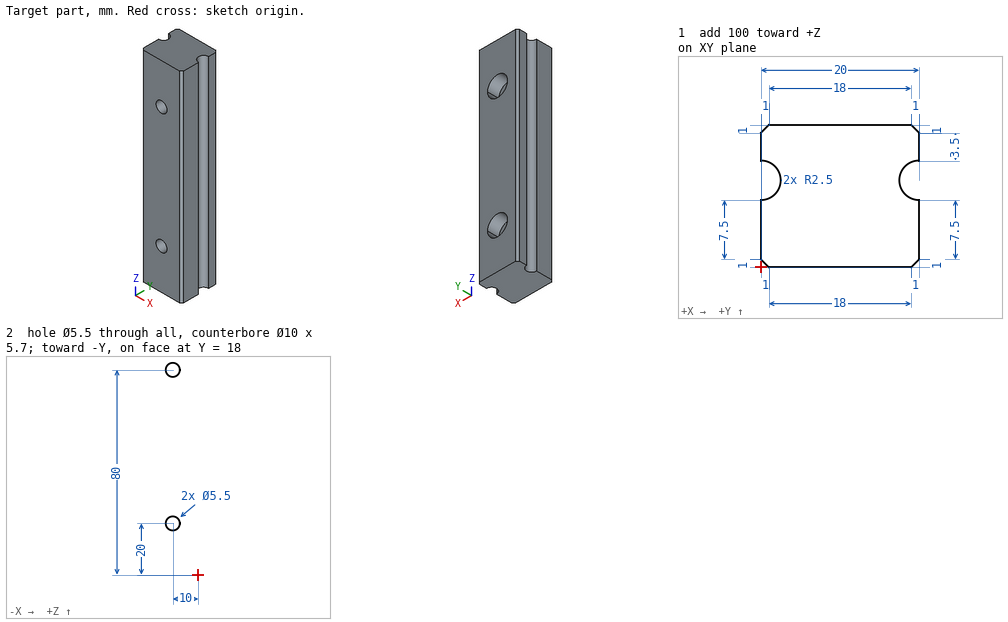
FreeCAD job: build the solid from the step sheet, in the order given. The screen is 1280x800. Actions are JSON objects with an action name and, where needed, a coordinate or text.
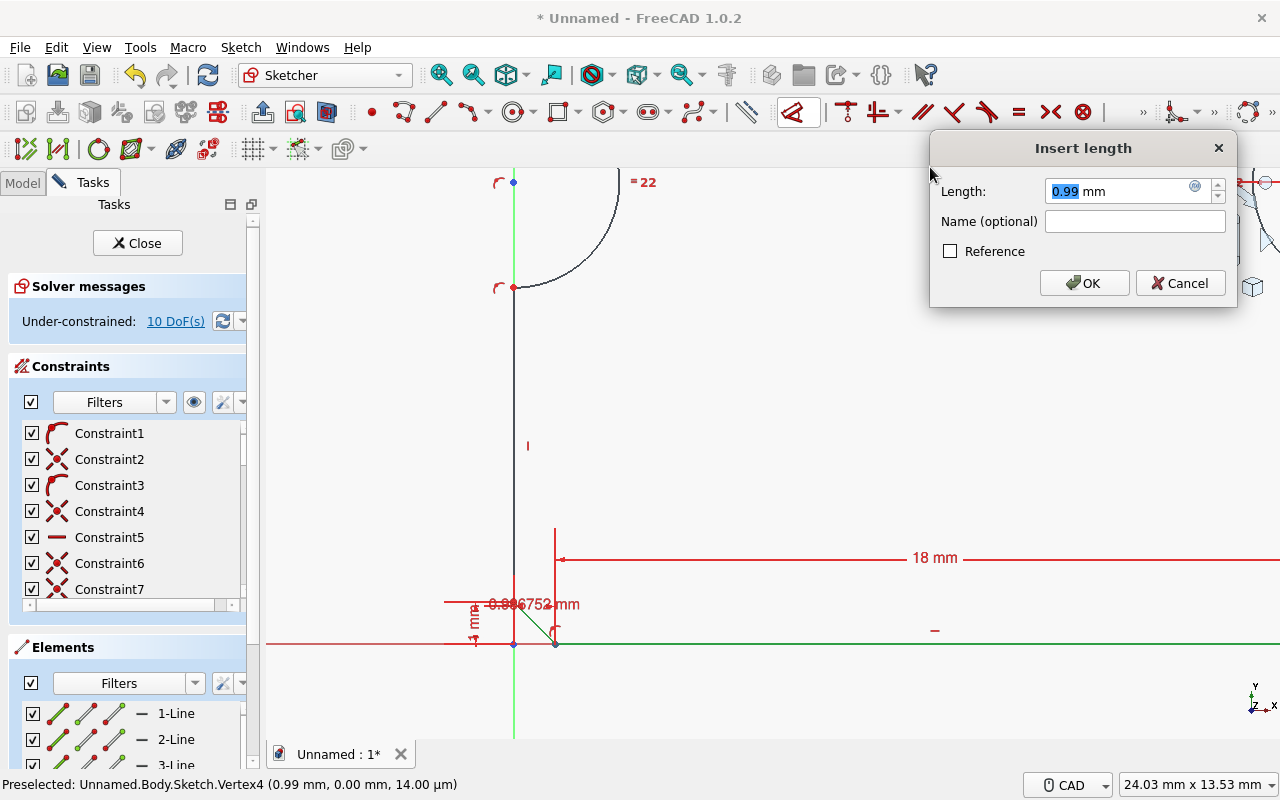
{"action": "type", "text": "1"}
{"action": "key", "text": "Return"}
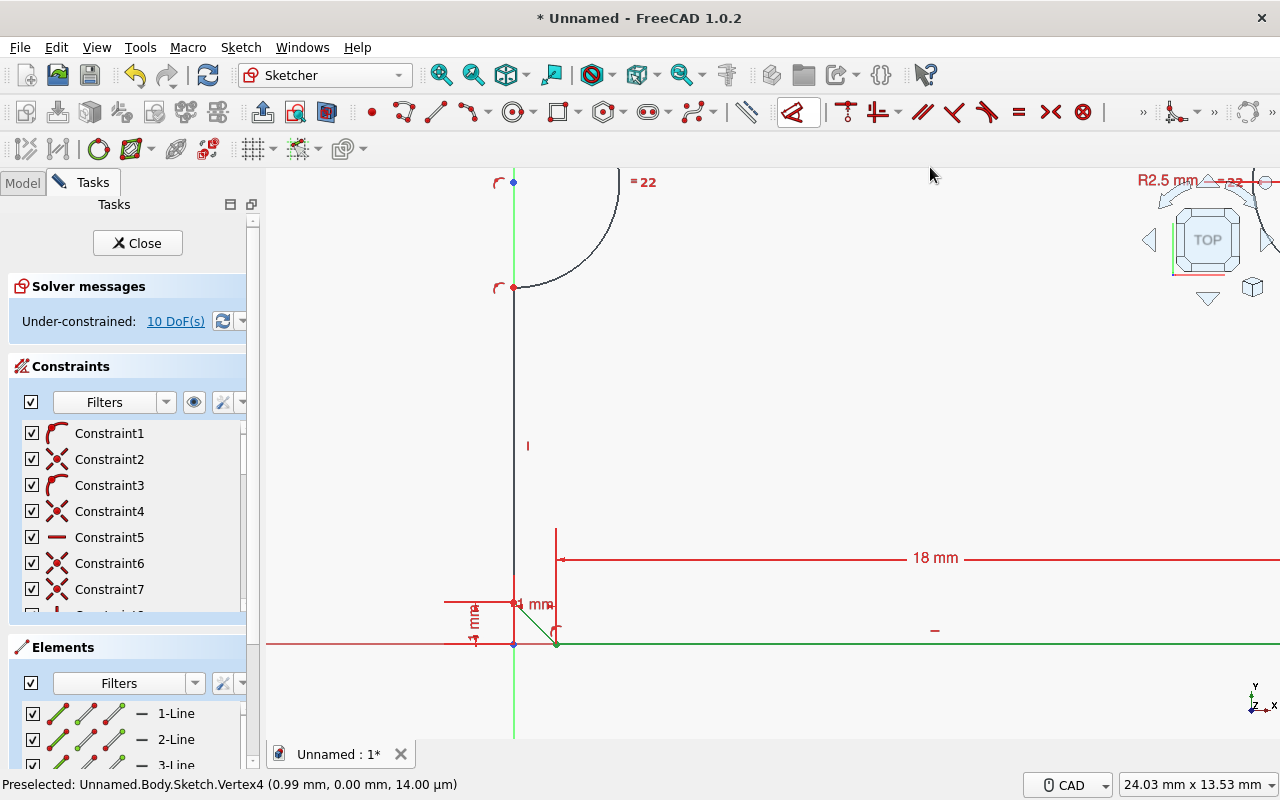
{"action": "scroll", "coordinate": [516, 608], "scroll_direction": "down", "scroll_amount": 4}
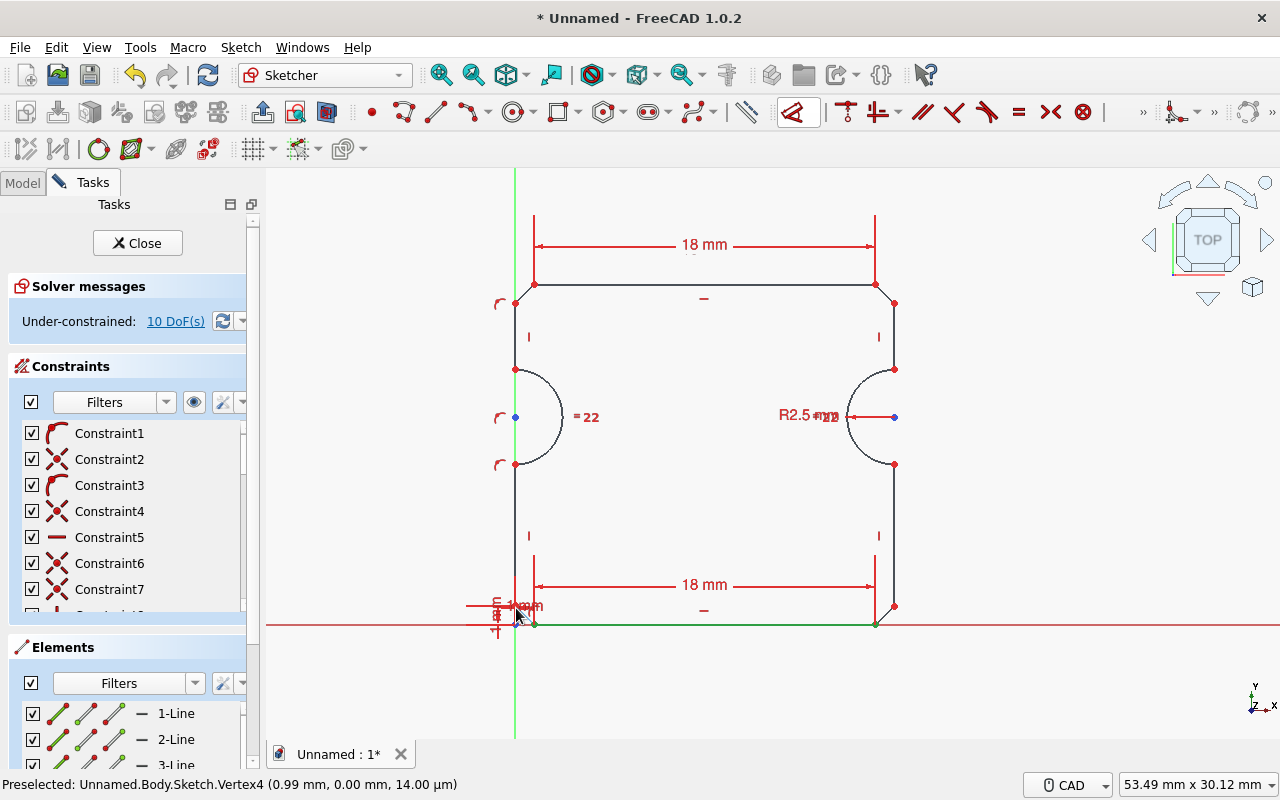
{"action": "scroll", "coordinate": [894, 607], "scroll_direction": "up", "scroll_amount": 4}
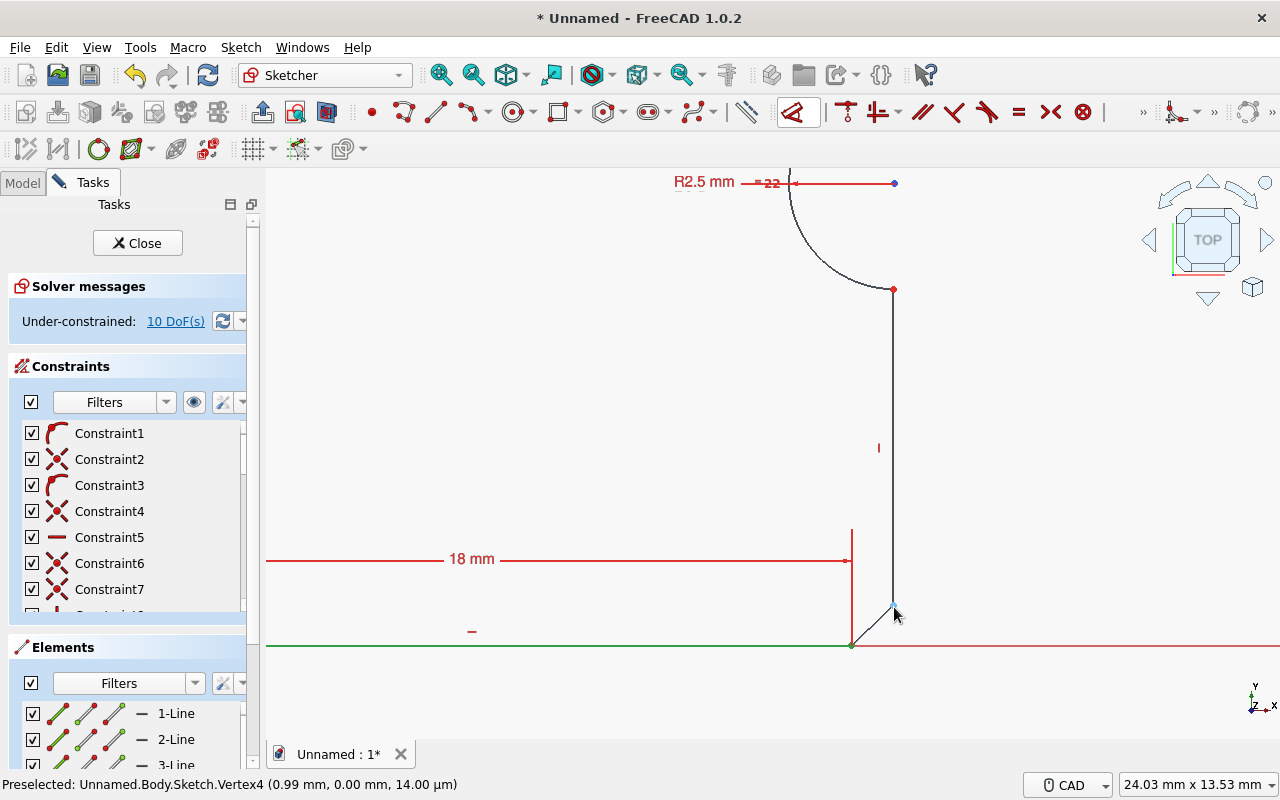
{"action": "left_click", "coordinate": [893, 605]}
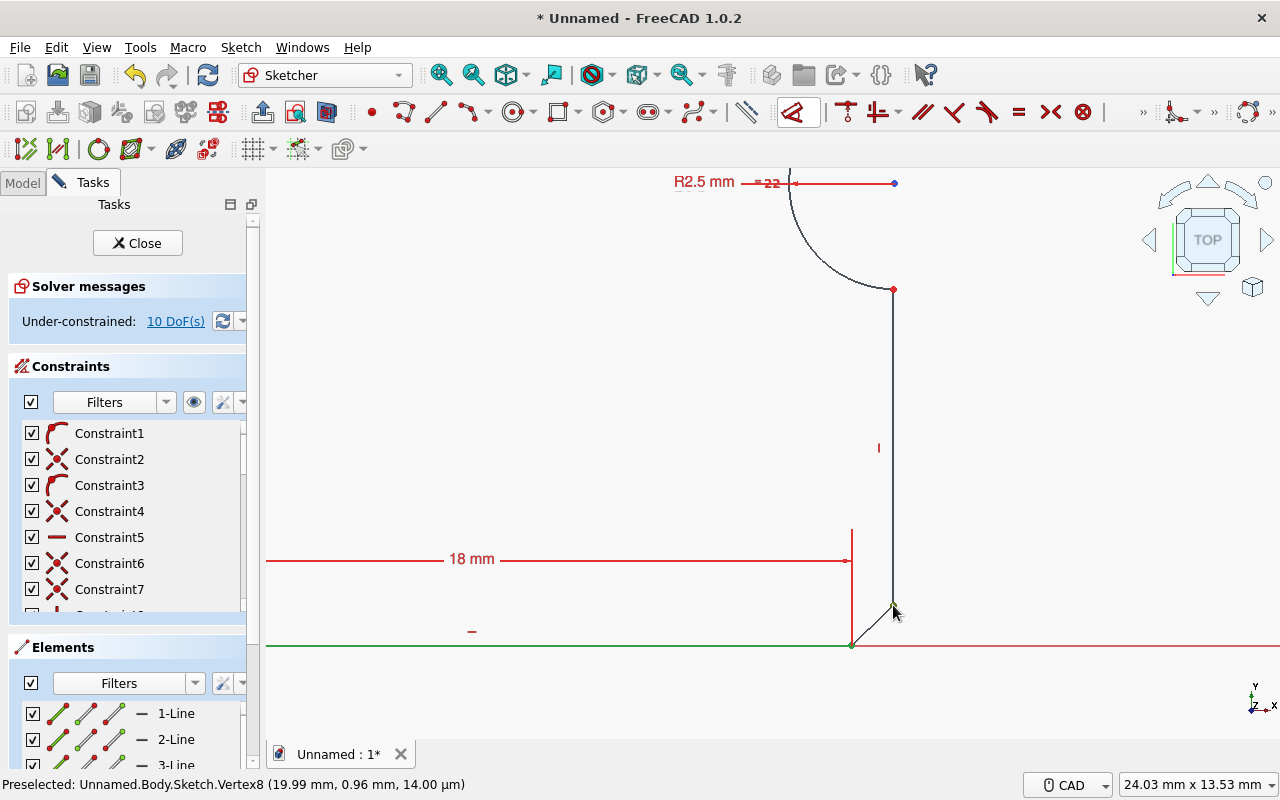
{"action": "left_click", "coordinate": [814, 112]}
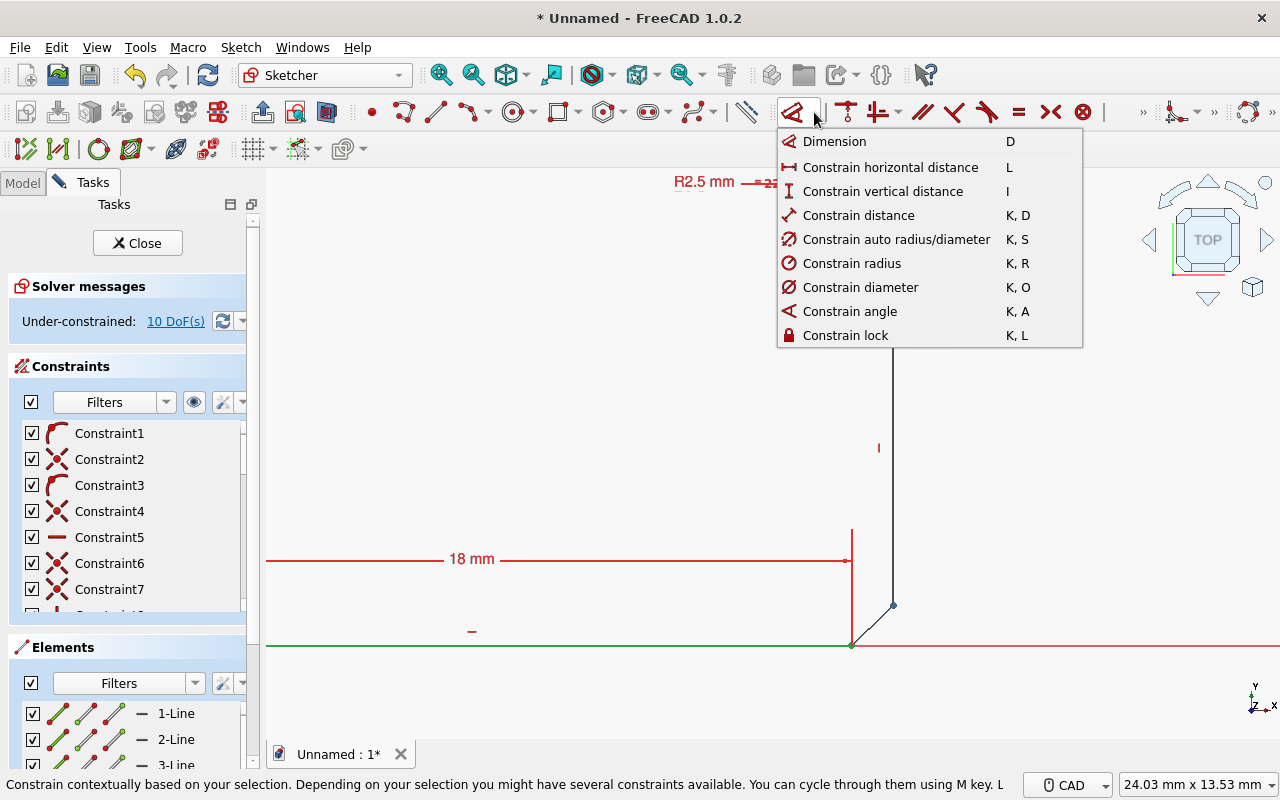
{"action": "left_click", "coordinate": [930, 191]}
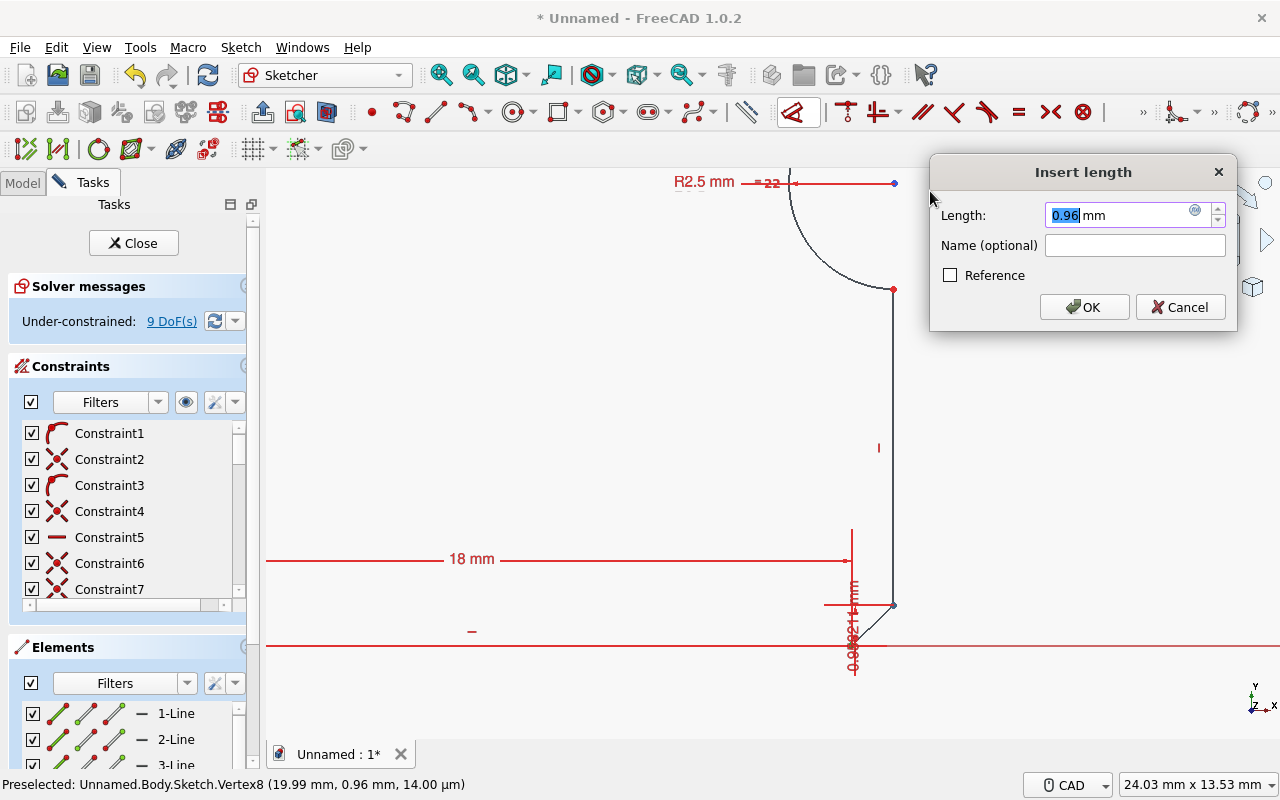
{"action": "type", "text": "1"}
{"action": "key", "text": "Return"}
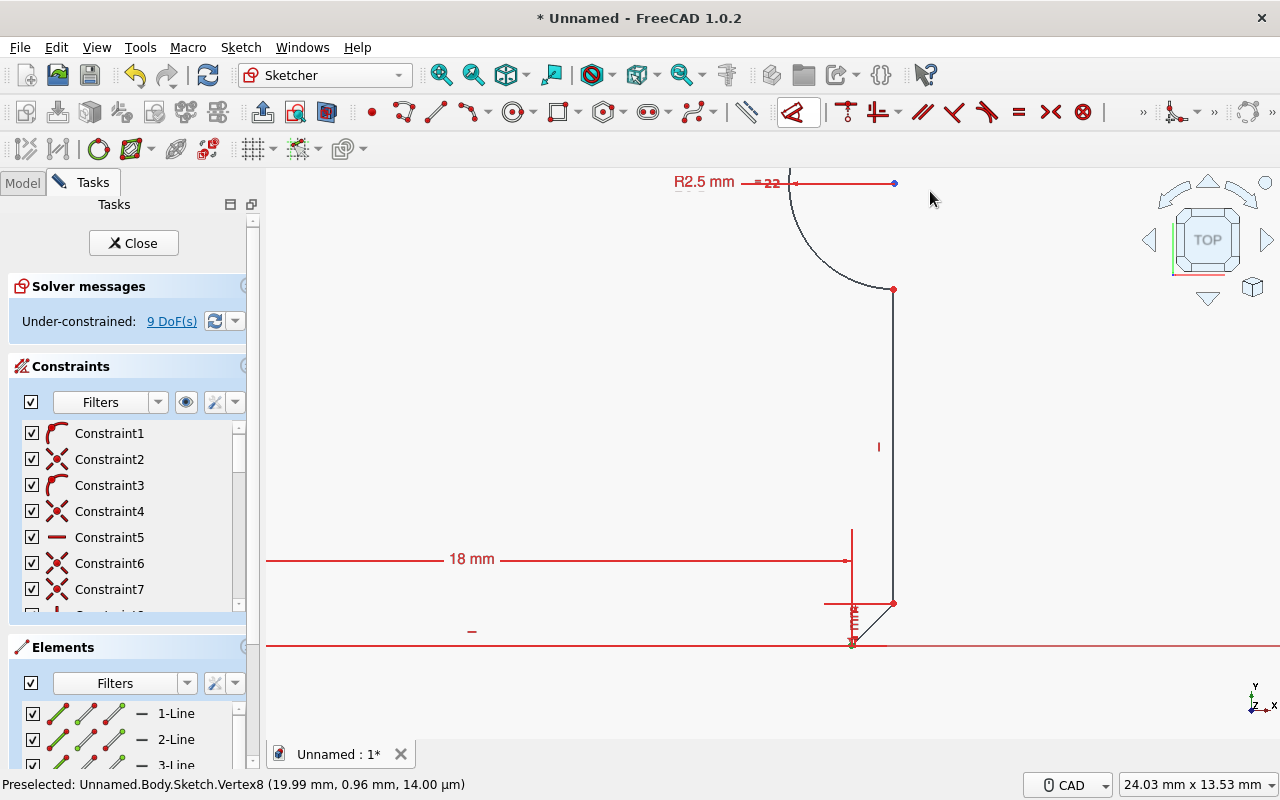
{"action": "scroll", "coordinate": [894, 606], "scroll_direction": "down", "scroll_amount": 4}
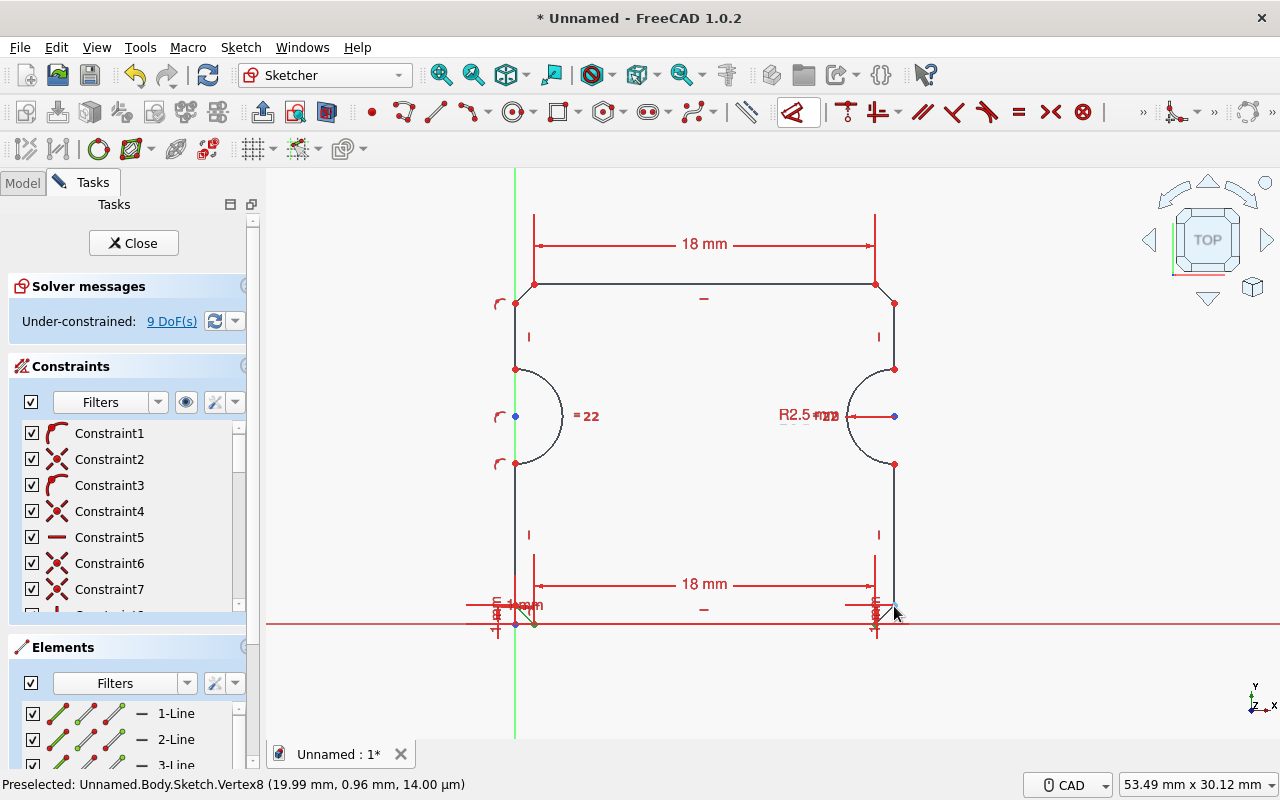
{"action": "scroll", "coordinate": [534, 284], "scroll_direction": "up", "scroll_amount": 4}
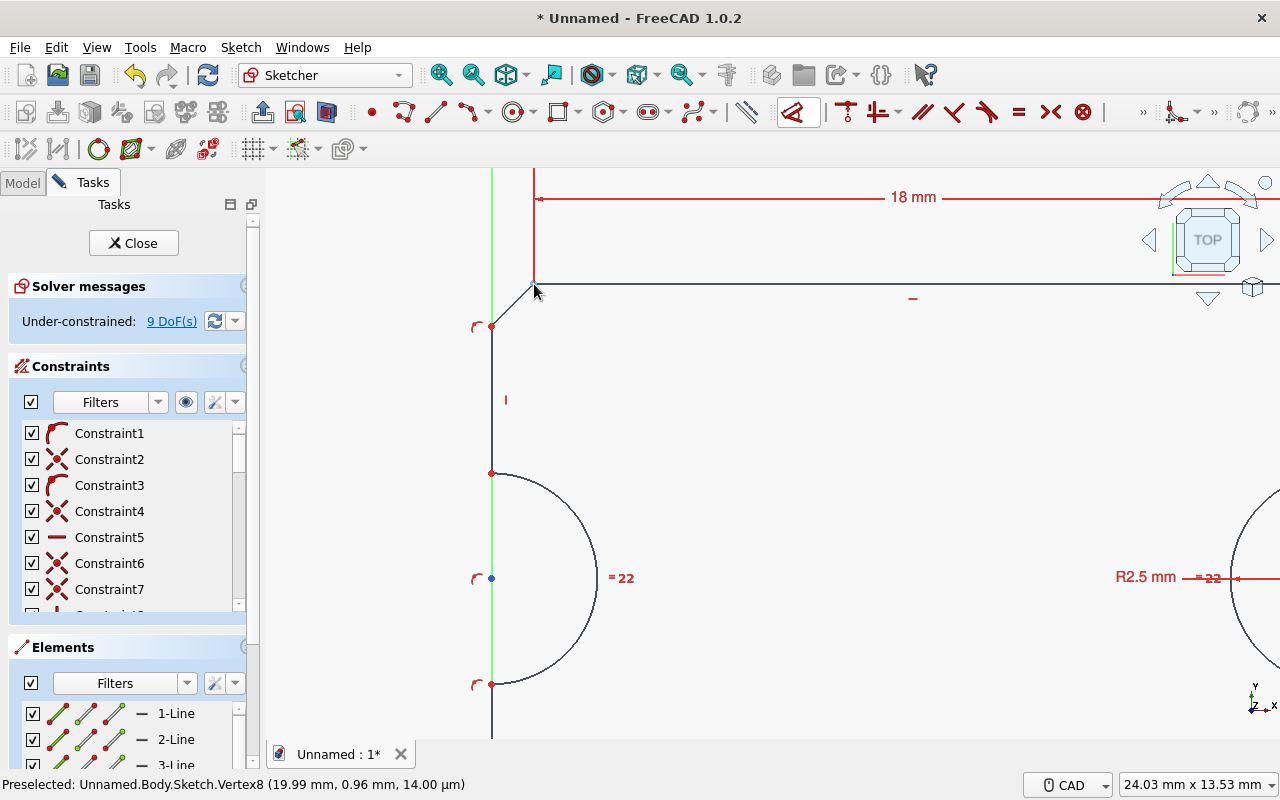
{"action": "left_click", "coordinate": [534, 284]}